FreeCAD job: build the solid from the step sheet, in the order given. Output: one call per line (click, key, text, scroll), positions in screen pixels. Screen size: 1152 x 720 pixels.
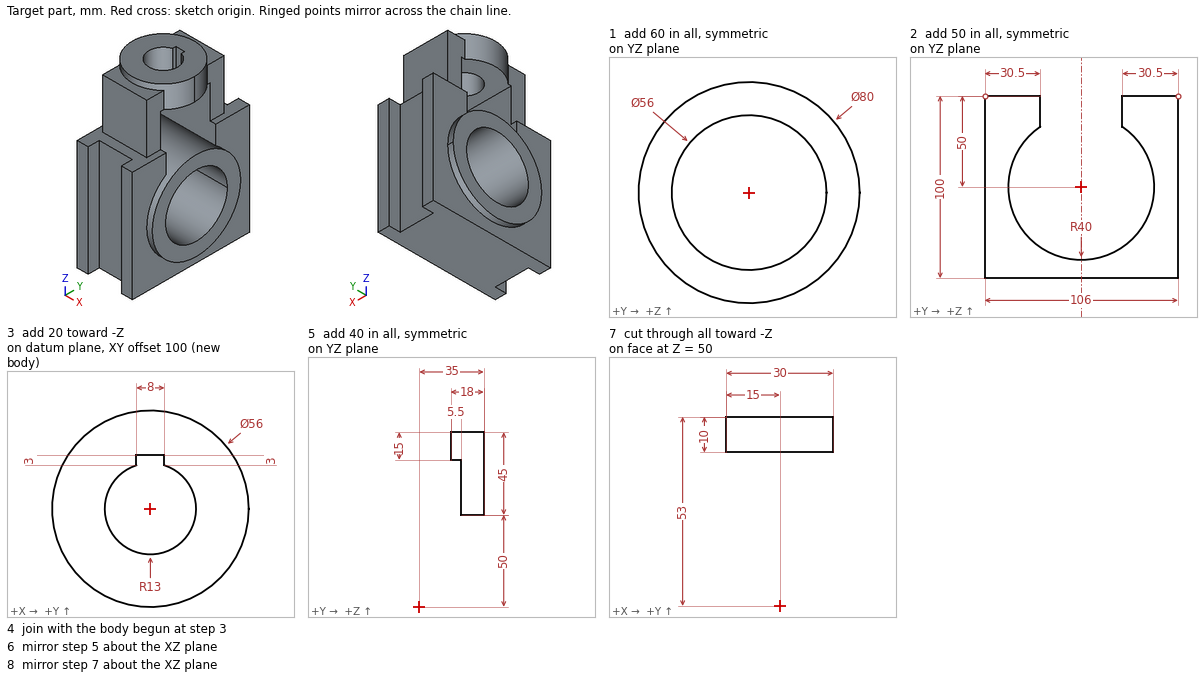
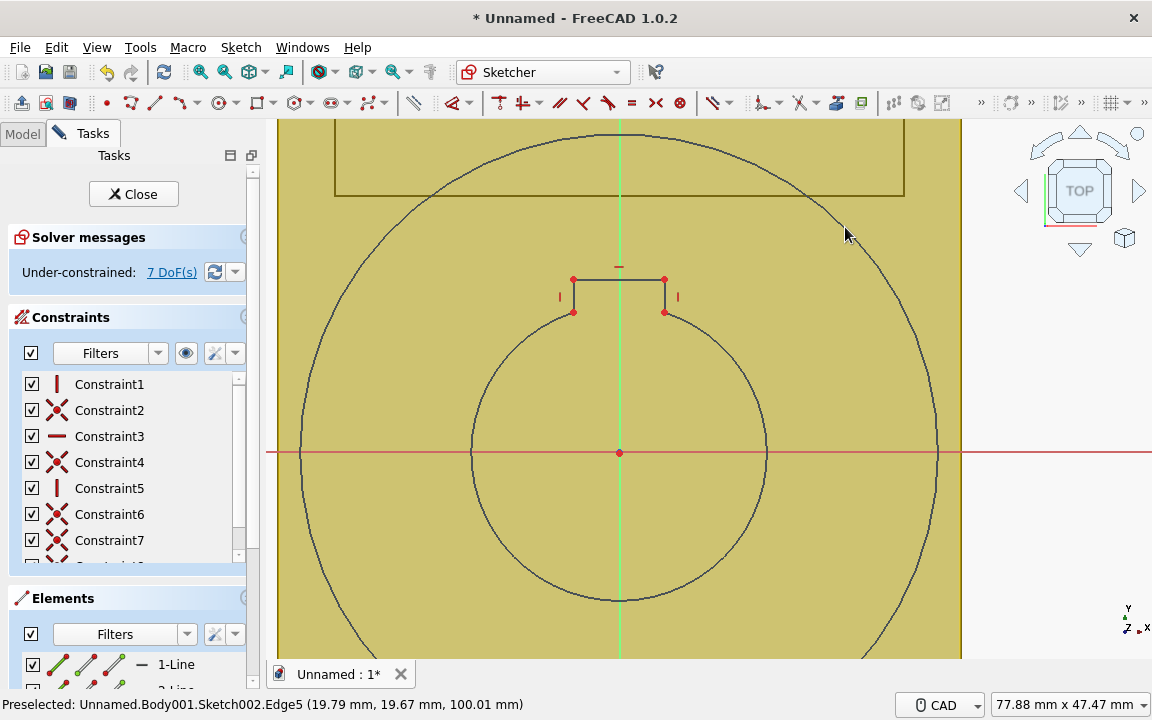
drag(609, 442, 630, 463)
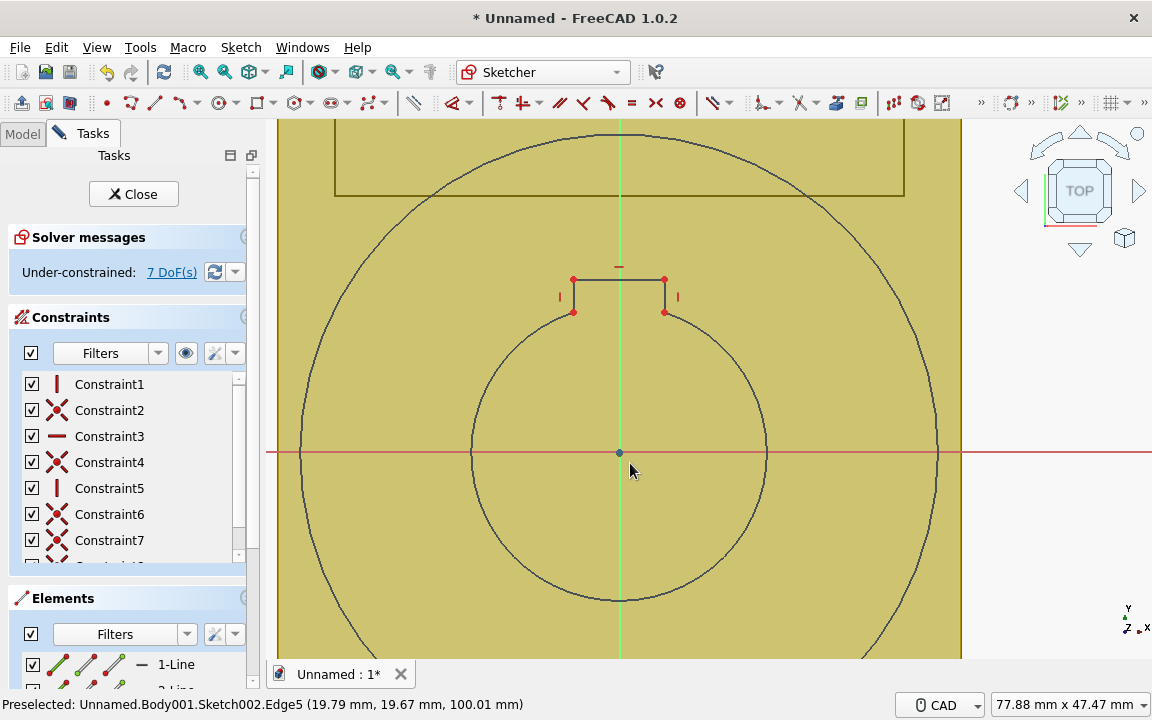
click(500, 104)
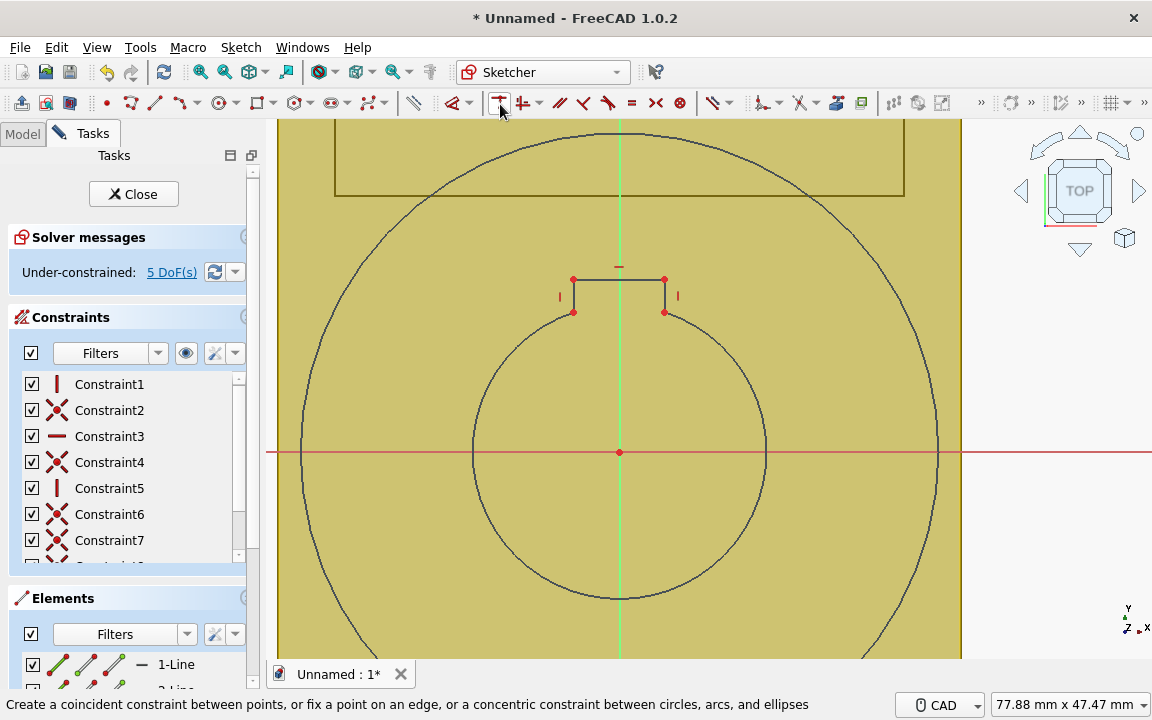
click(452, 104)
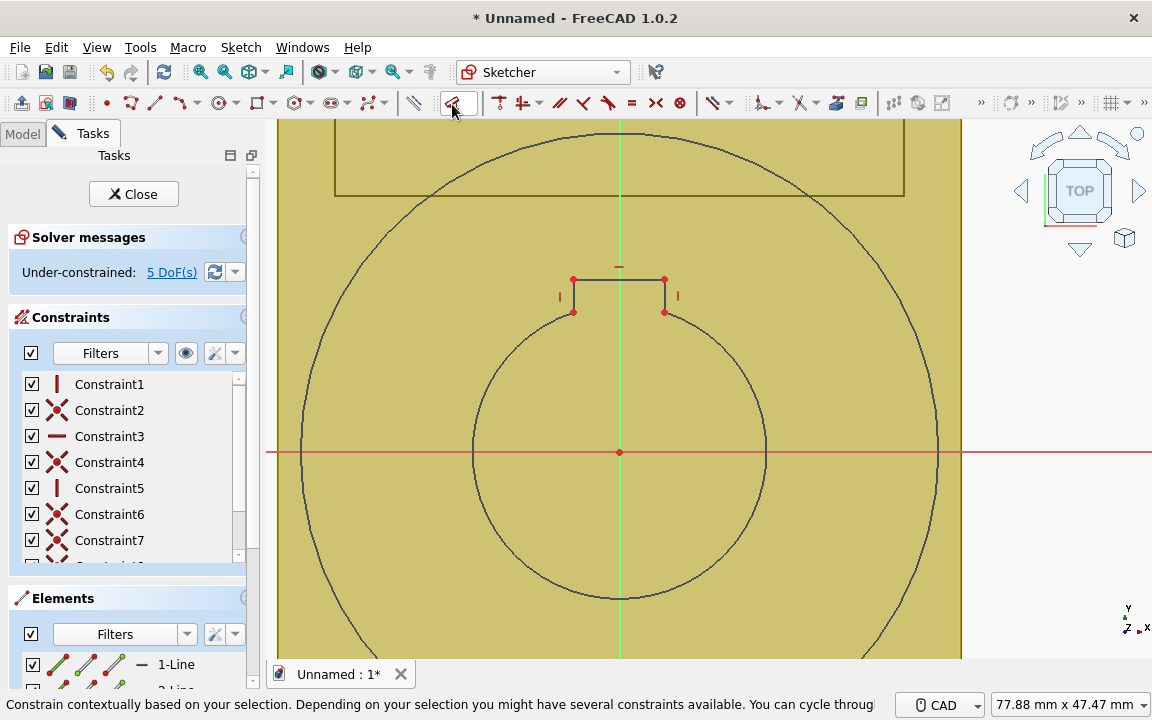
click(487, 515)
click(458, 529)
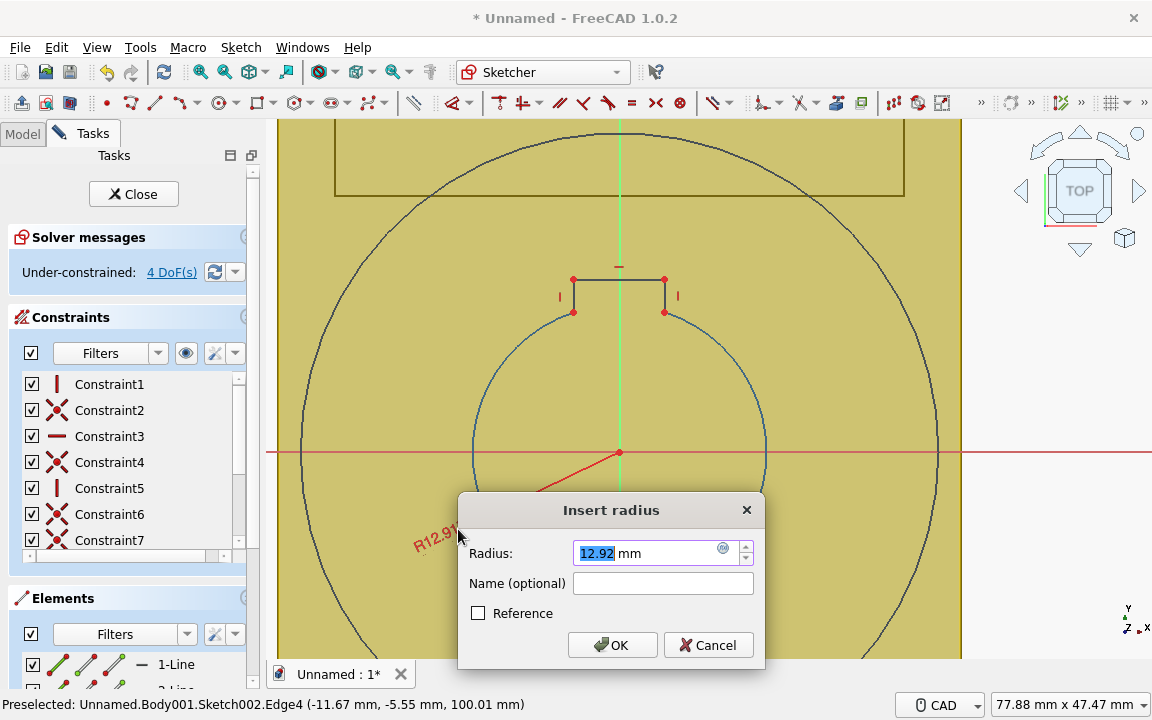
text(13)
key(Return)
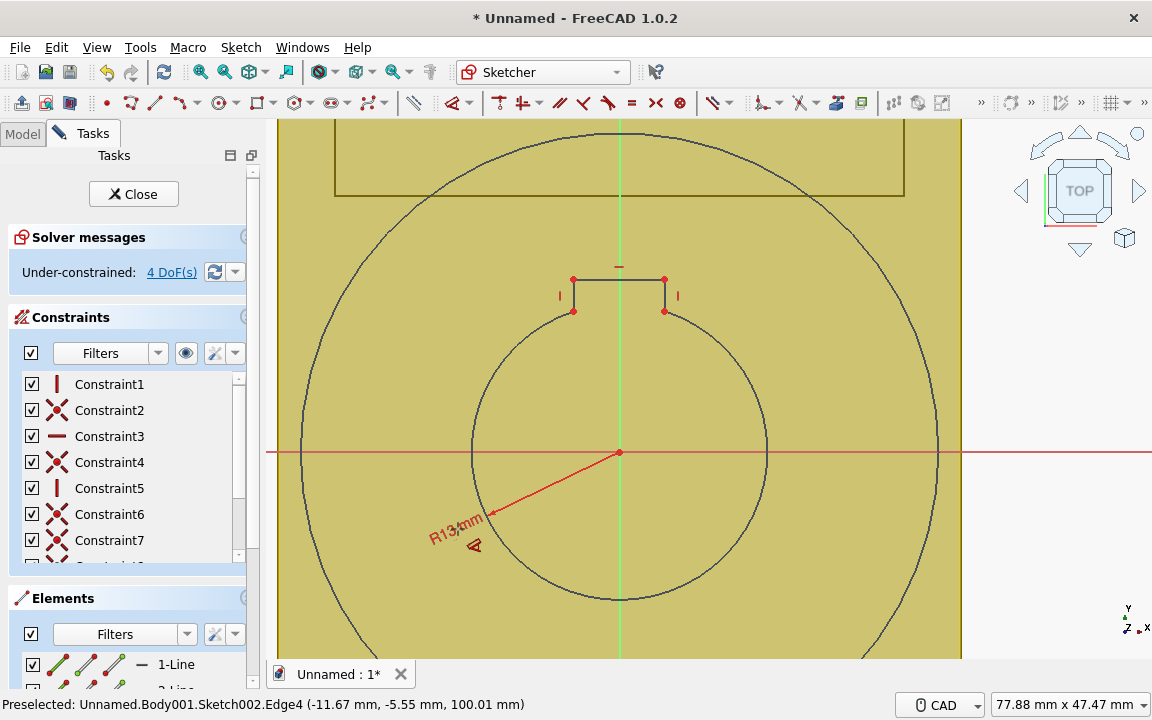
click(844, 226)
click(867, 203)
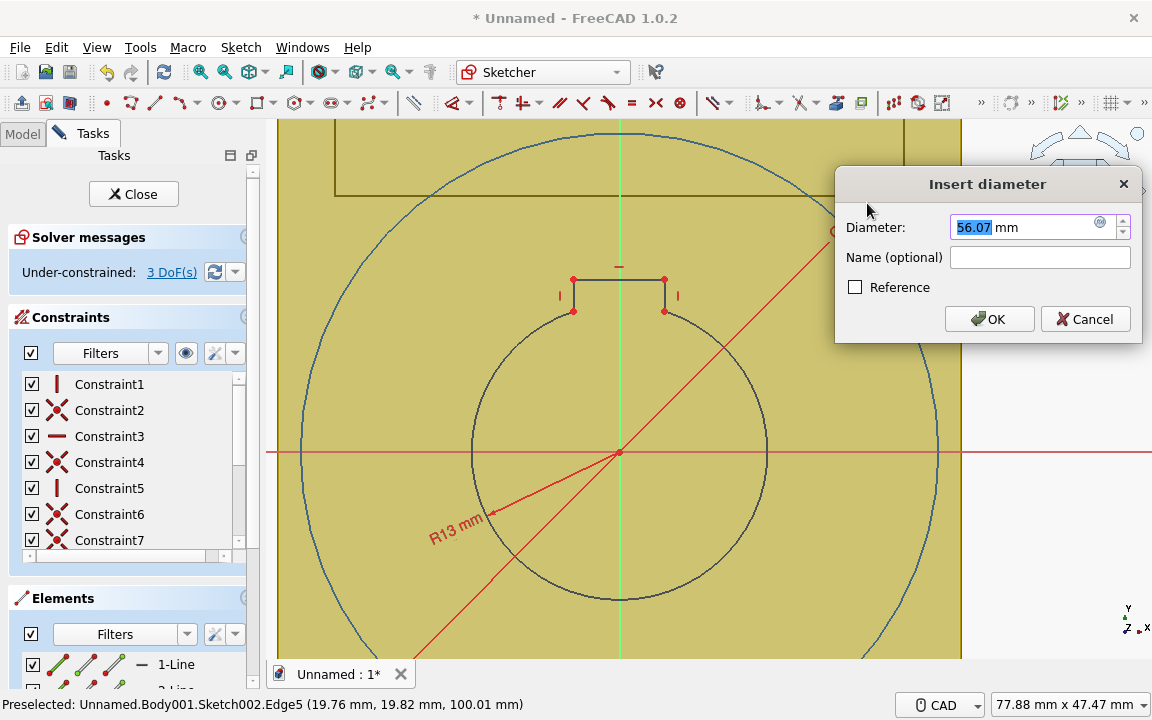
text(56)
key(Return)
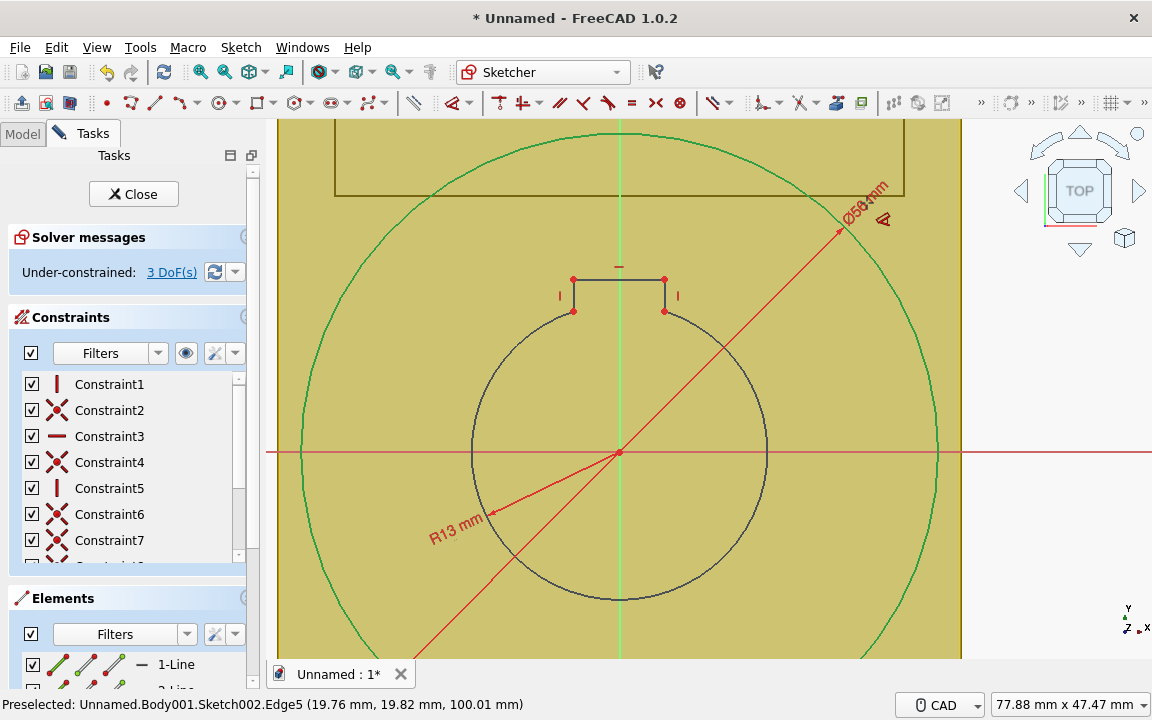
scroll(574, 302, up, 2)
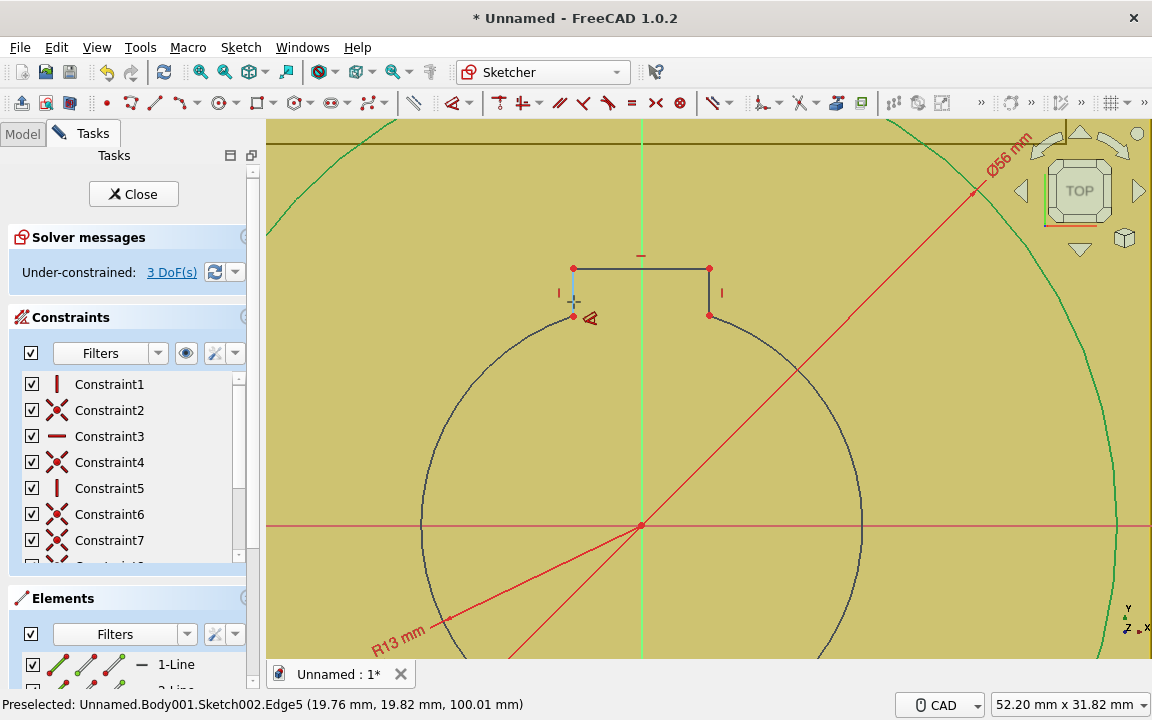
click(573, 302)
click(539, 292)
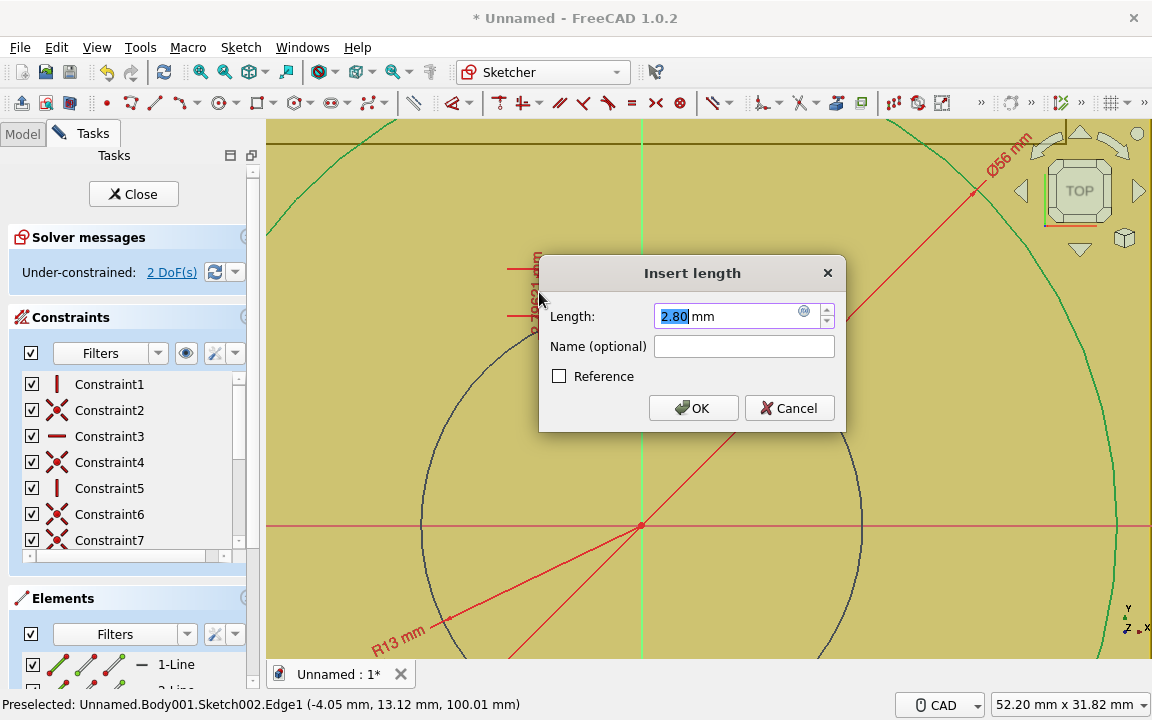
text(3)
key(Return)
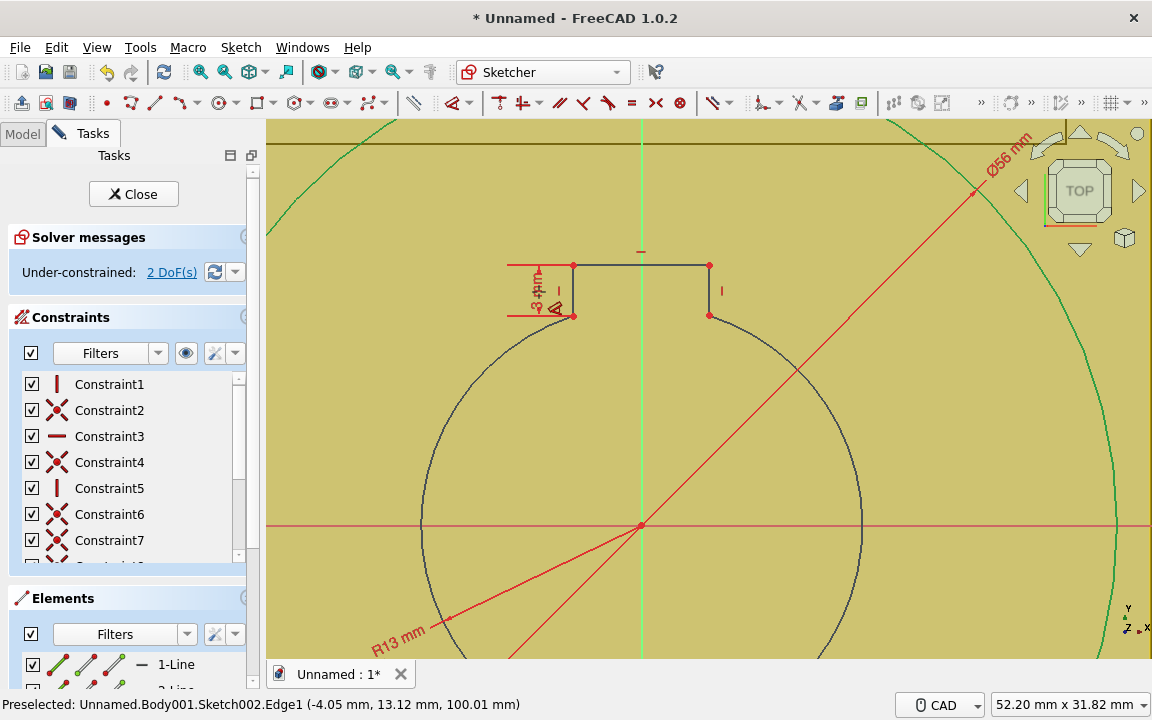
click(614, 265)
click(610, 231)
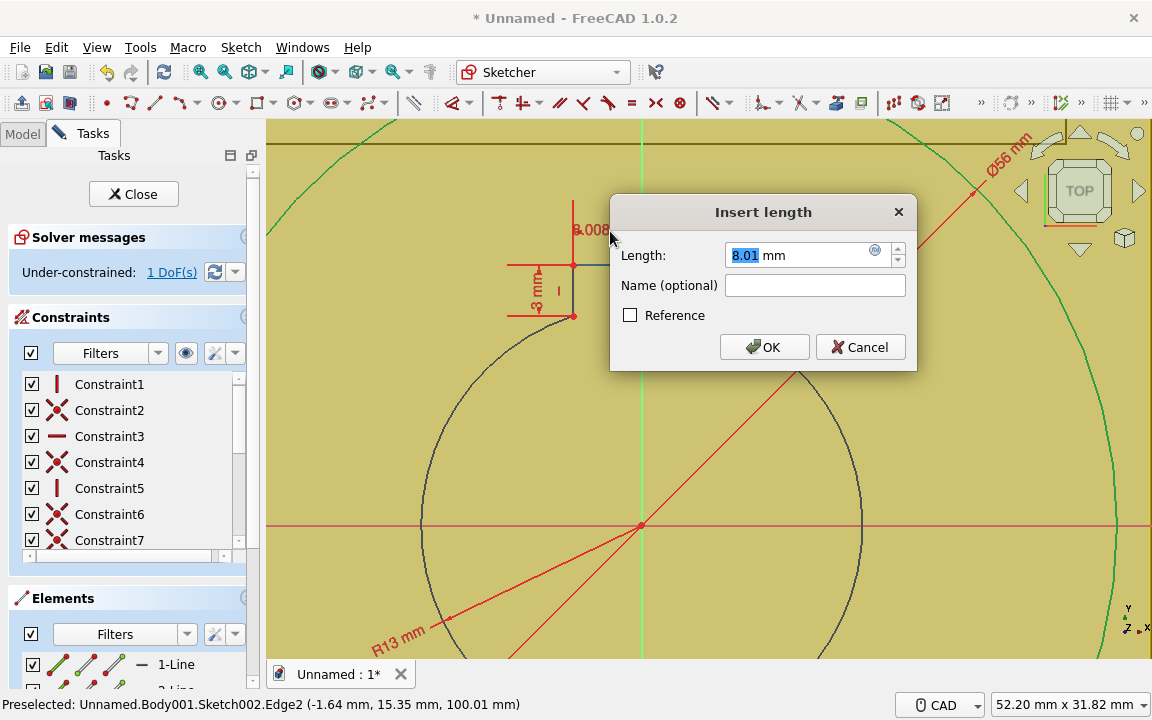
text(8)
key(Return)